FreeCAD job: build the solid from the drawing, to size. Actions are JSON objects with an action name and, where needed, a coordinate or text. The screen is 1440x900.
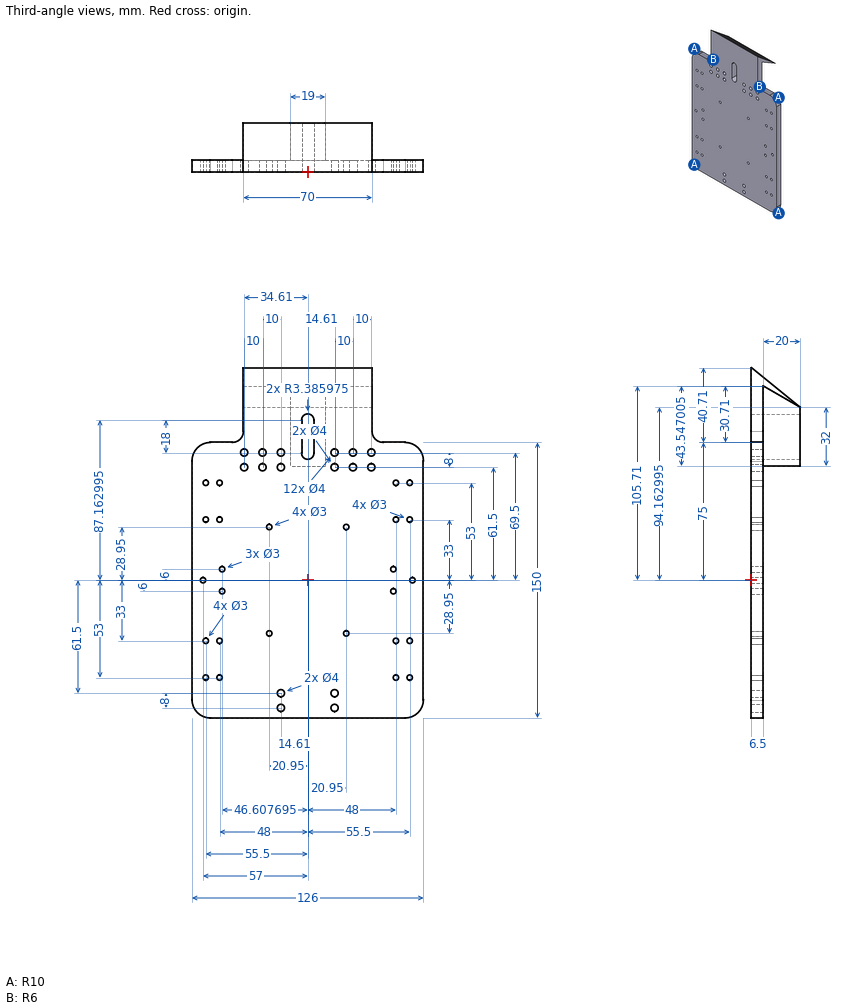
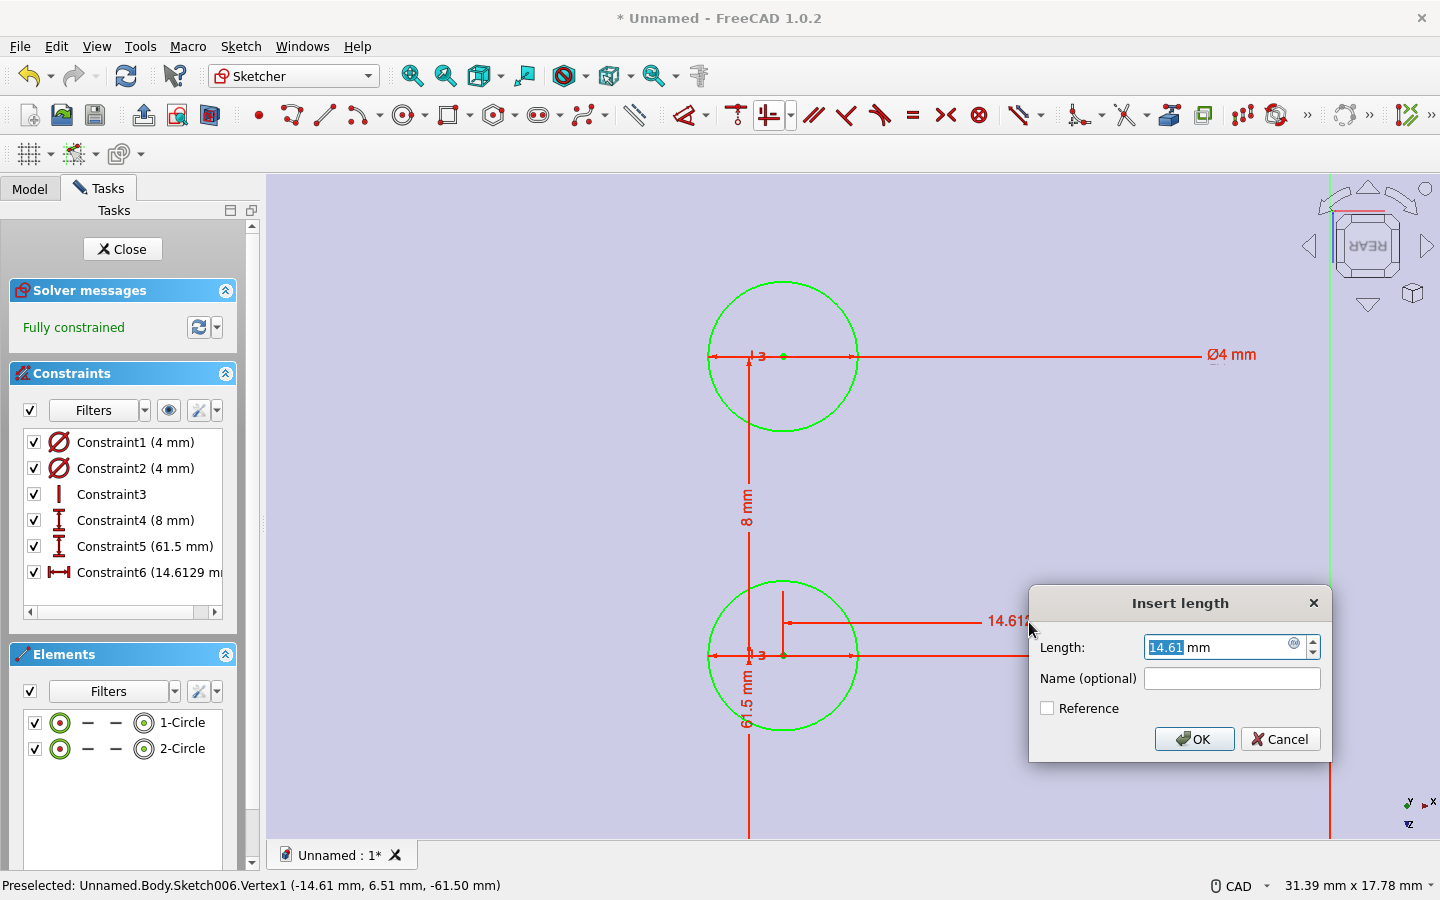
{"action": "type", "text": "14.61"}
{"action": "key", "text": "Return"}
{"action": "key", "text": "Escape"}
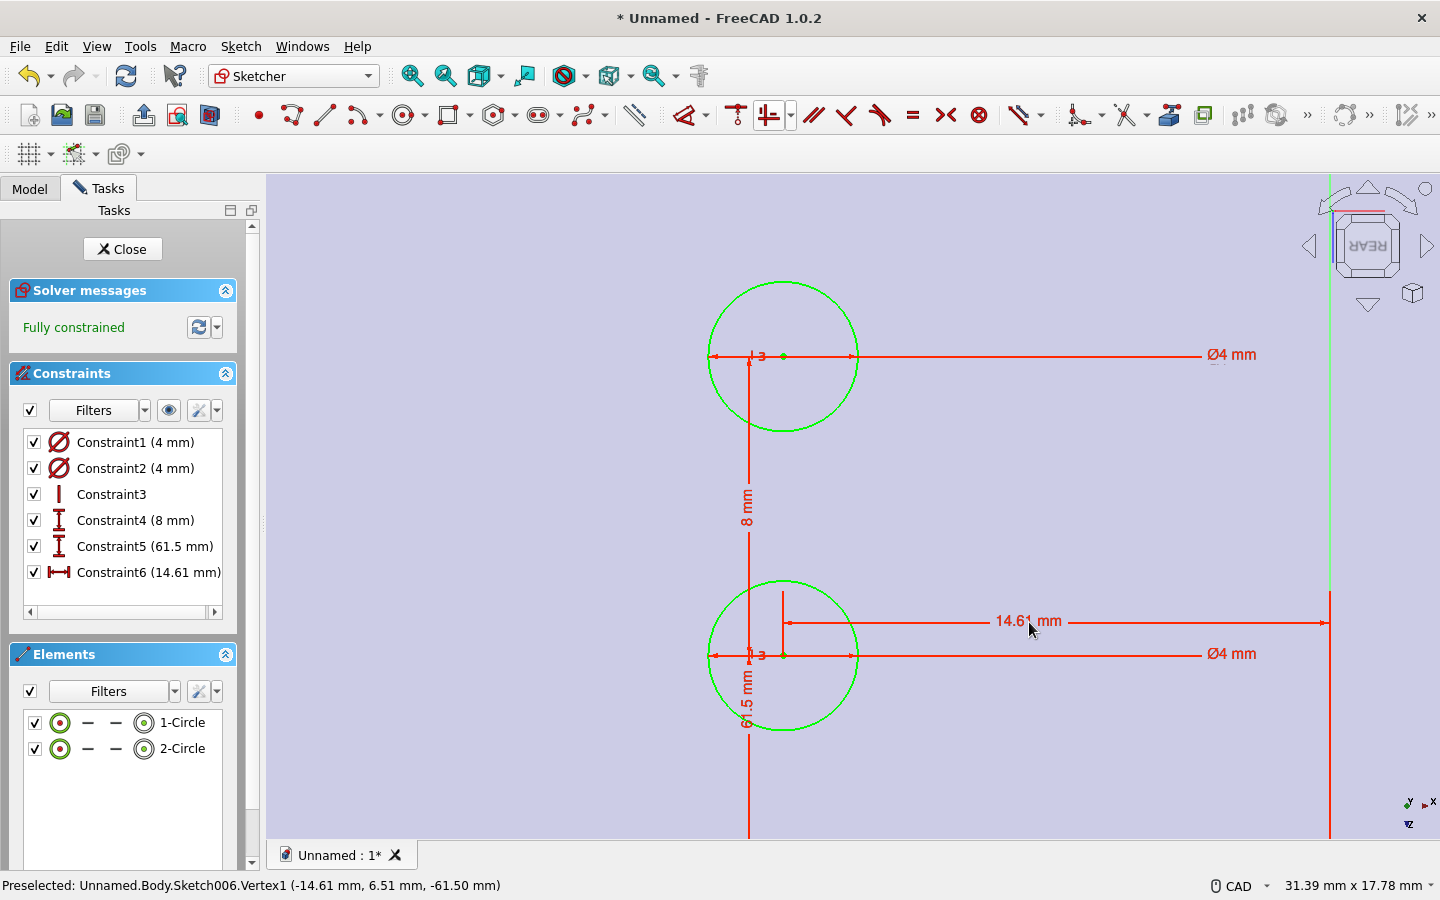
{"action": "left_click", "coordinate": [123, 249]}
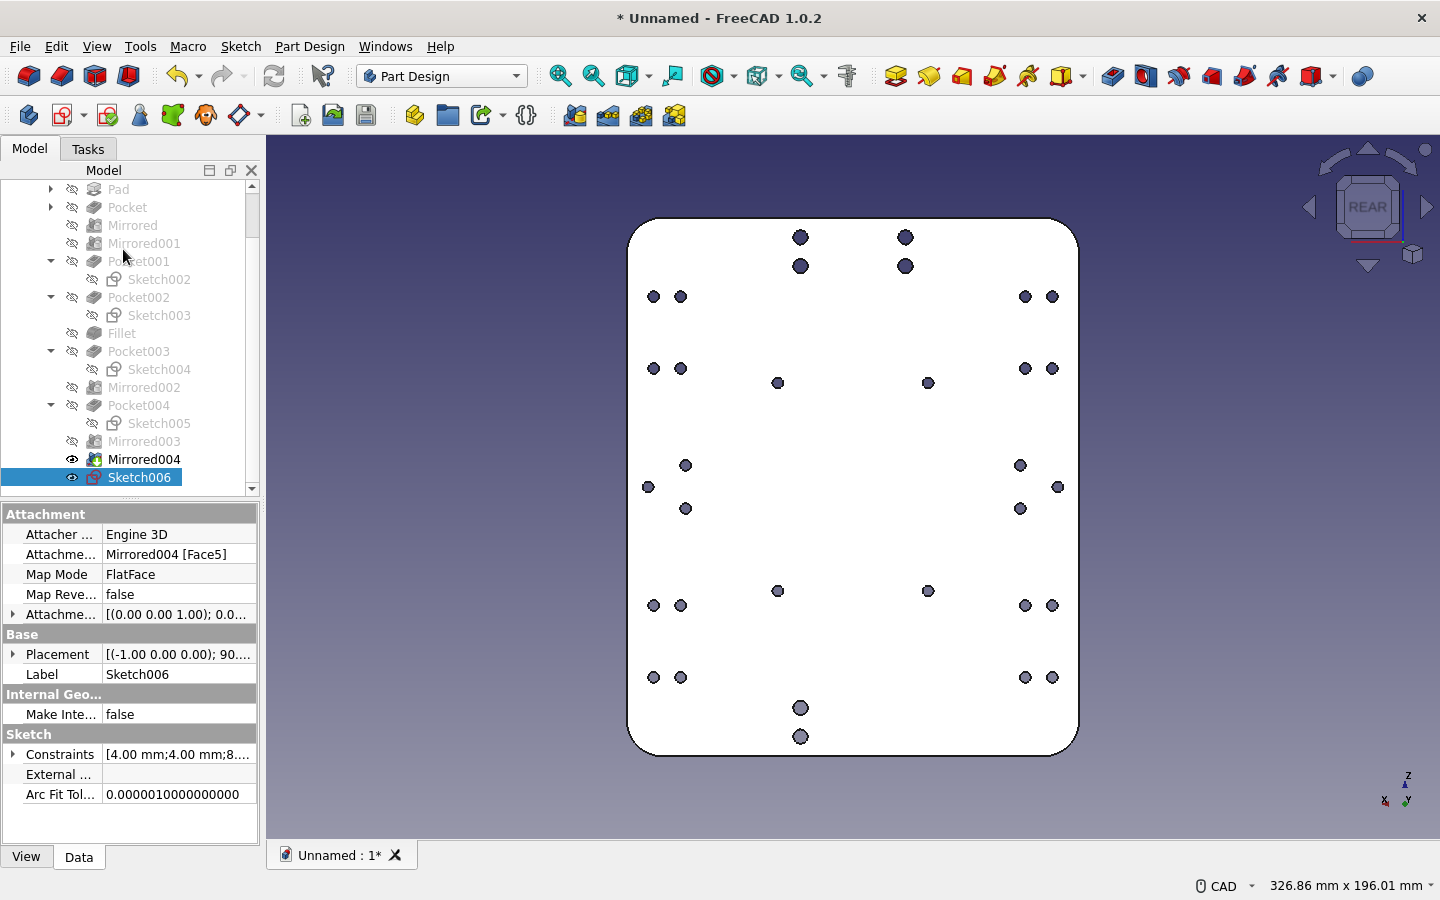
{"action": "left_click", "coordinate": [1113, 76]}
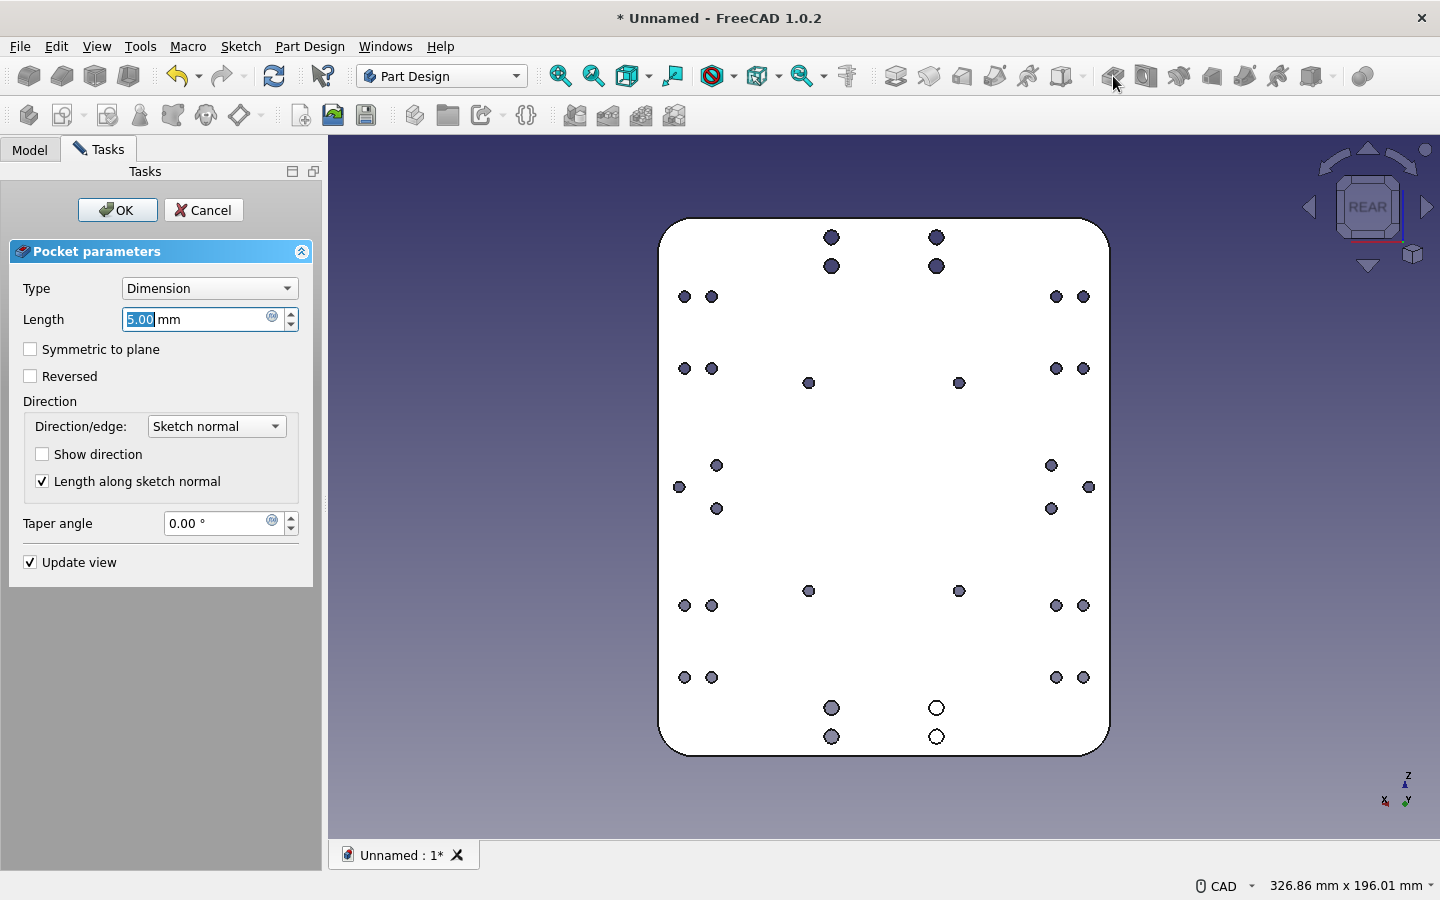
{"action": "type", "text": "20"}
{"action": "key", "text": "Tab"}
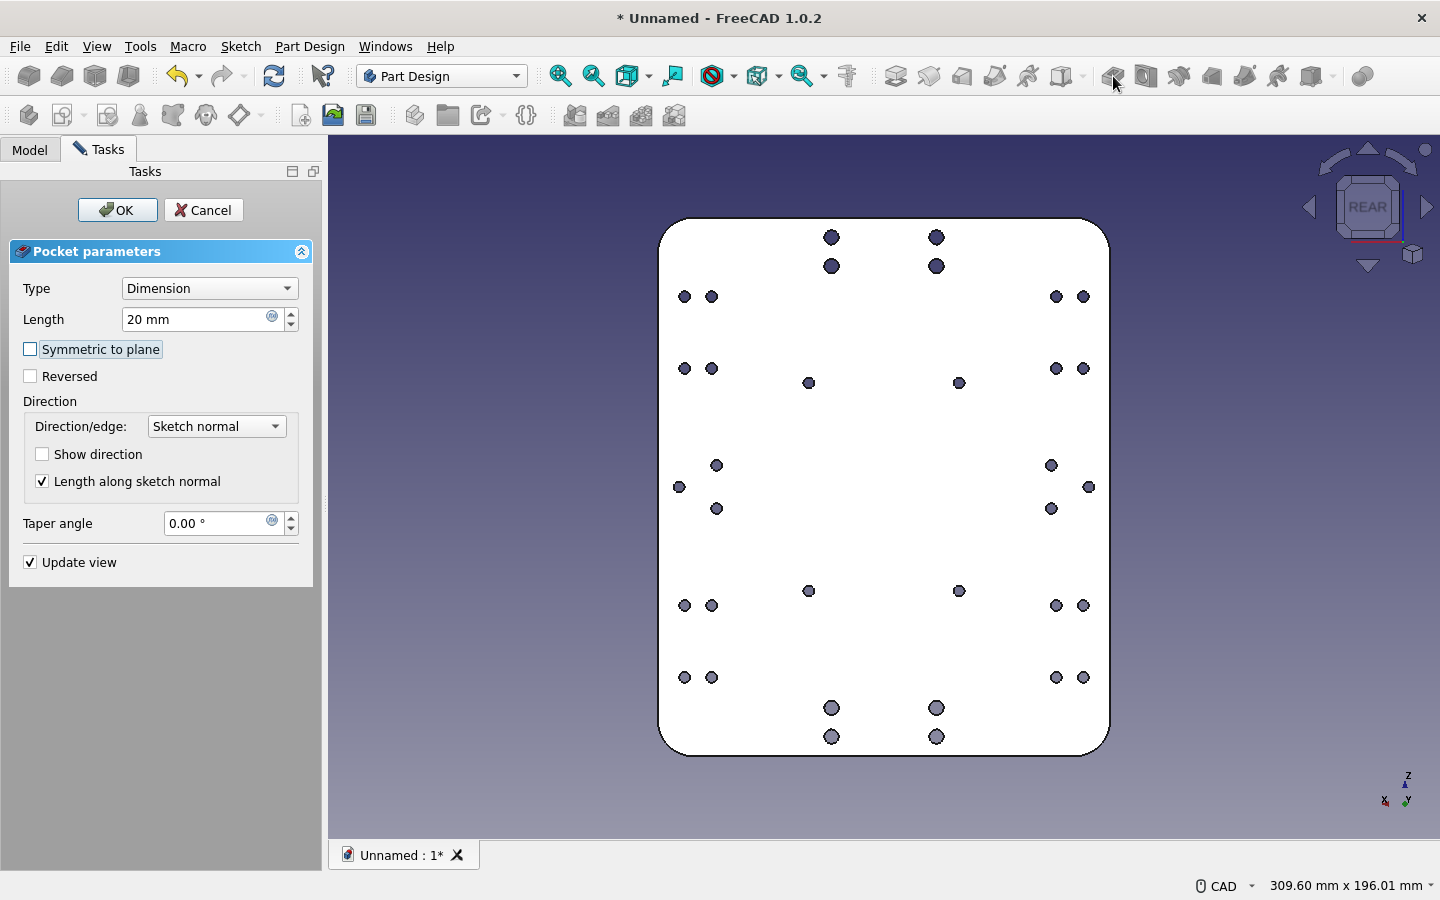
{"action": "left_click", "coordinate": [118, 210]}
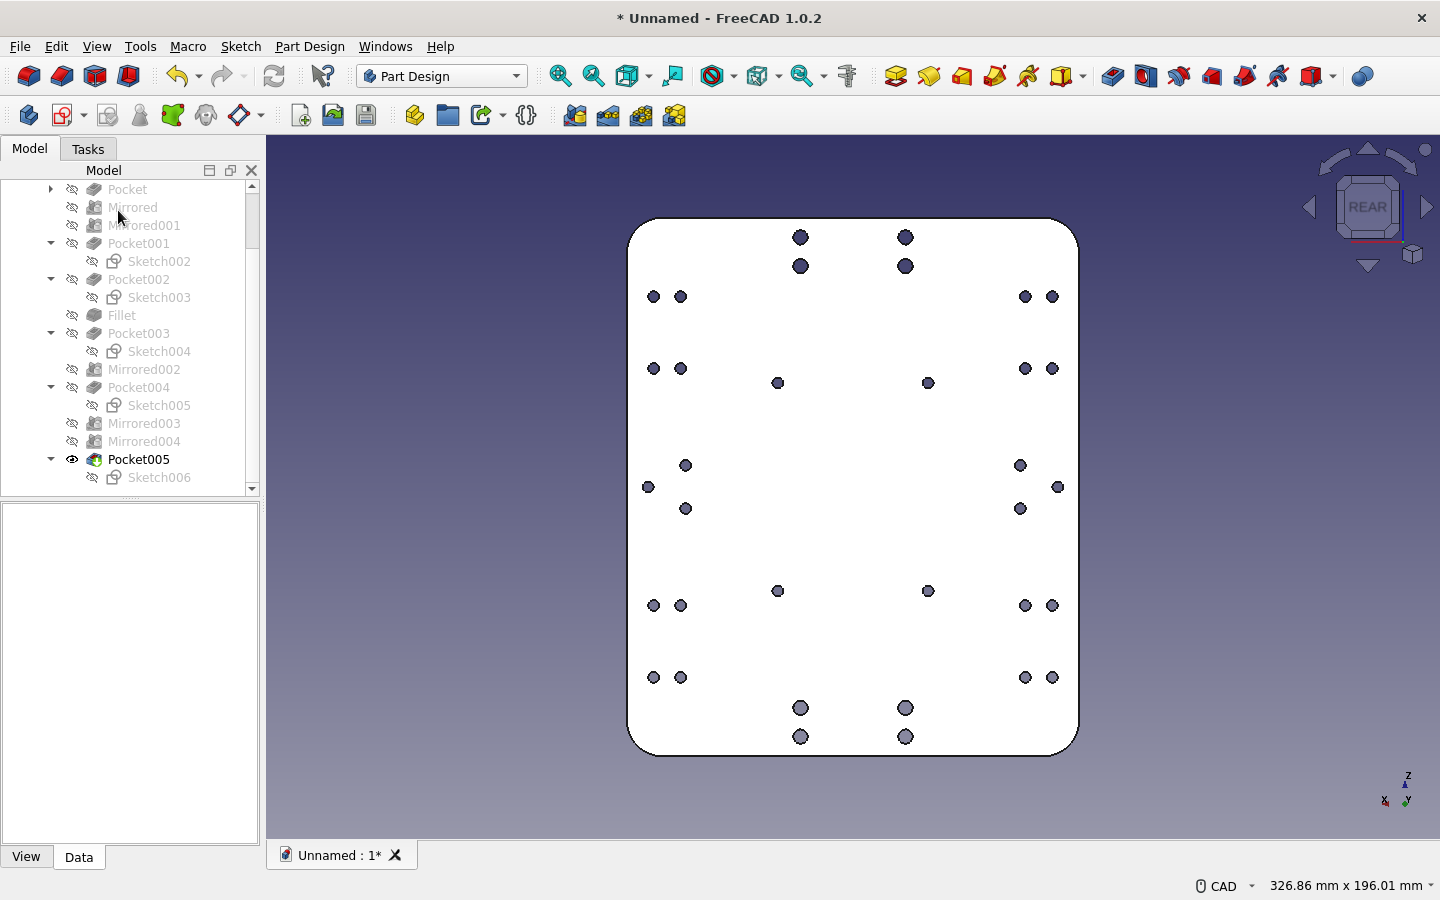
{"action": "left_click", "coordinate": [853, 486]}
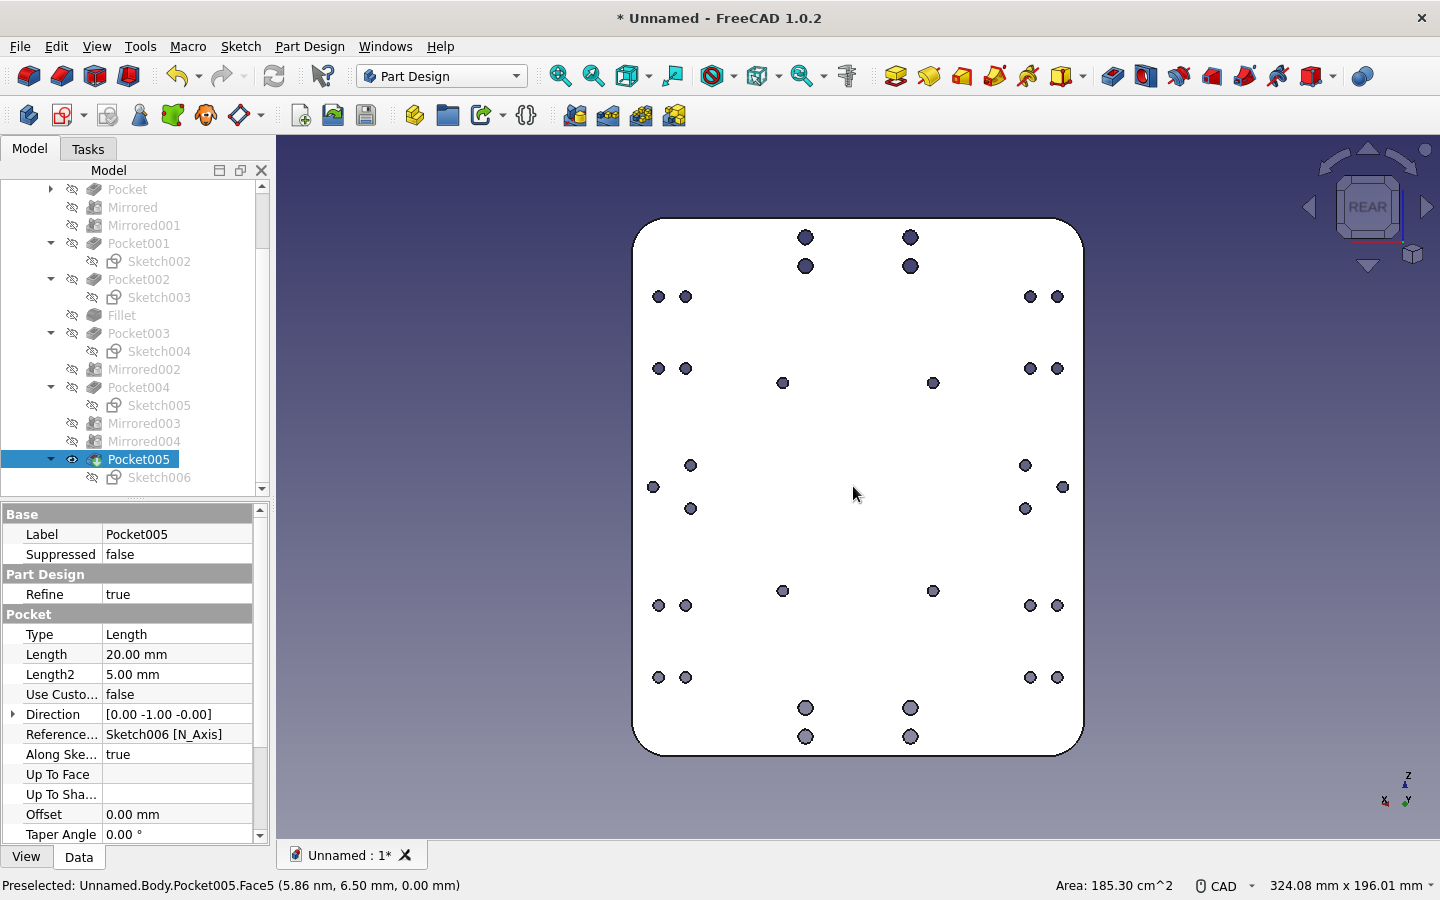
{"action": "left_click", "coordinate": [62, 116]}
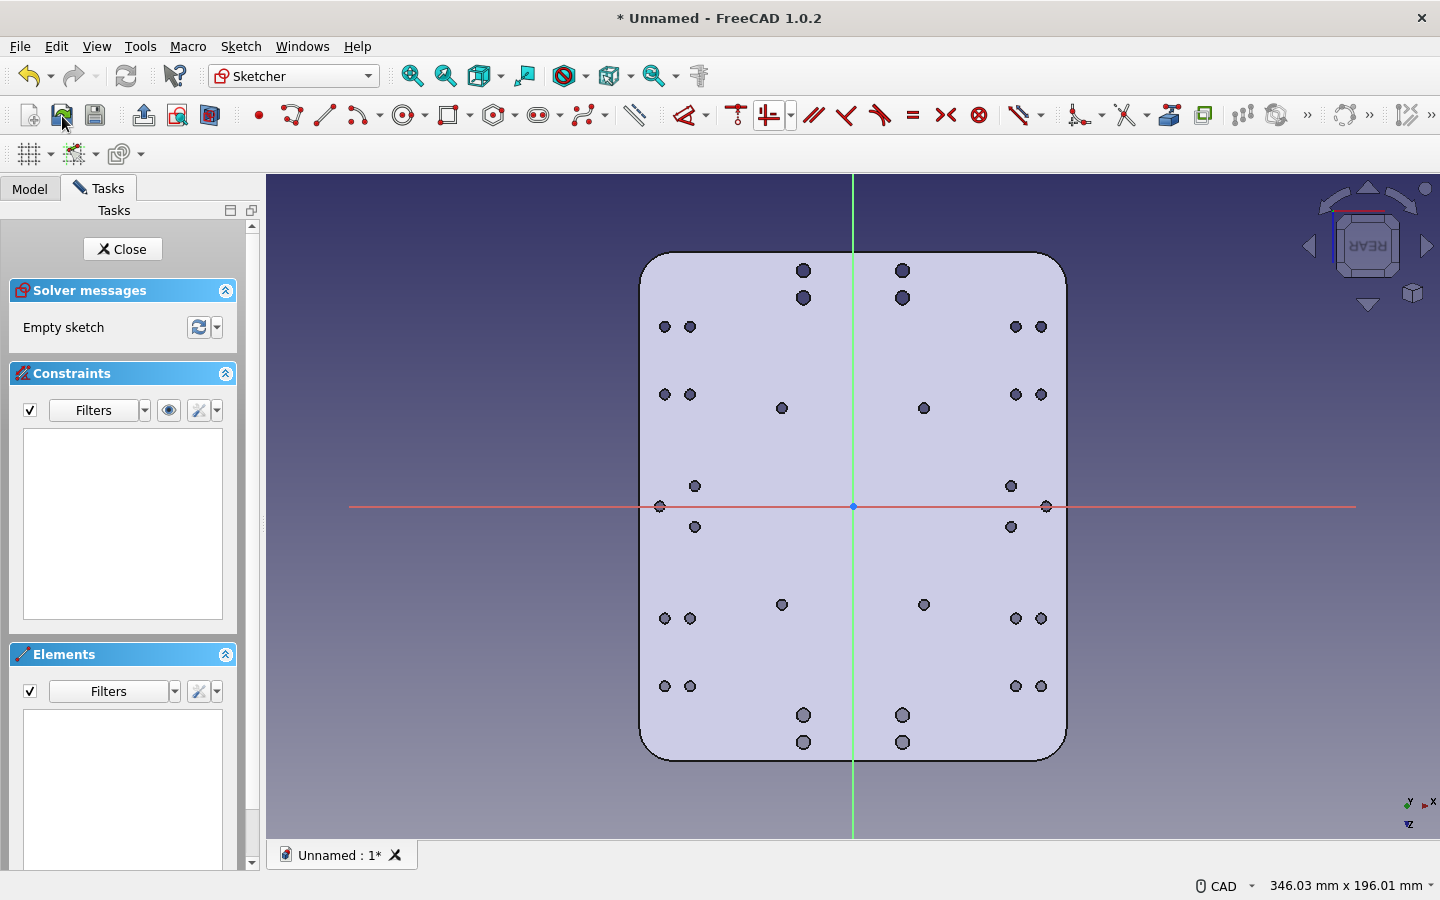
{"action": "scroll", "coordinate": [936, 775], "scroll_direction": "up", "scroll_amount": 3}